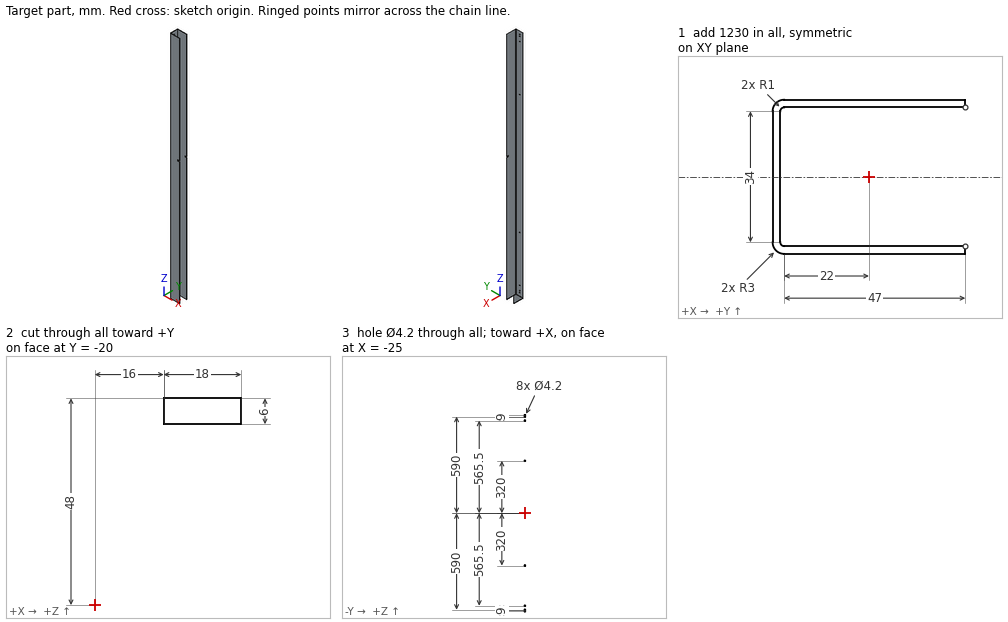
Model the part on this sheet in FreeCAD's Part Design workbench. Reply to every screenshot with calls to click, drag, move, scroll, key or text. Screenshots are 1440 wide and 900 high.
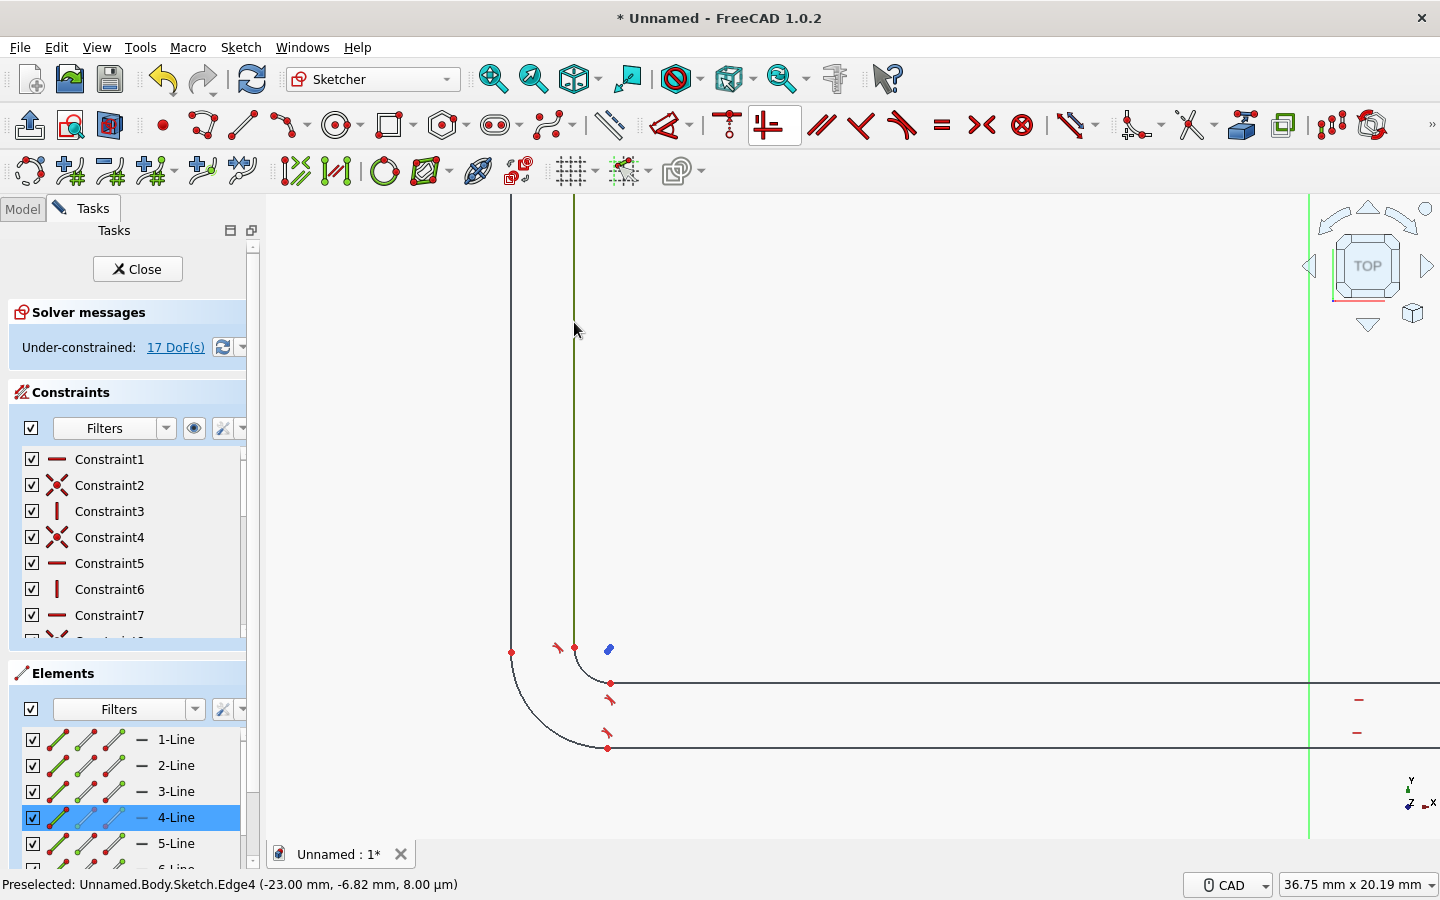
scroll(558, 694, down, 6)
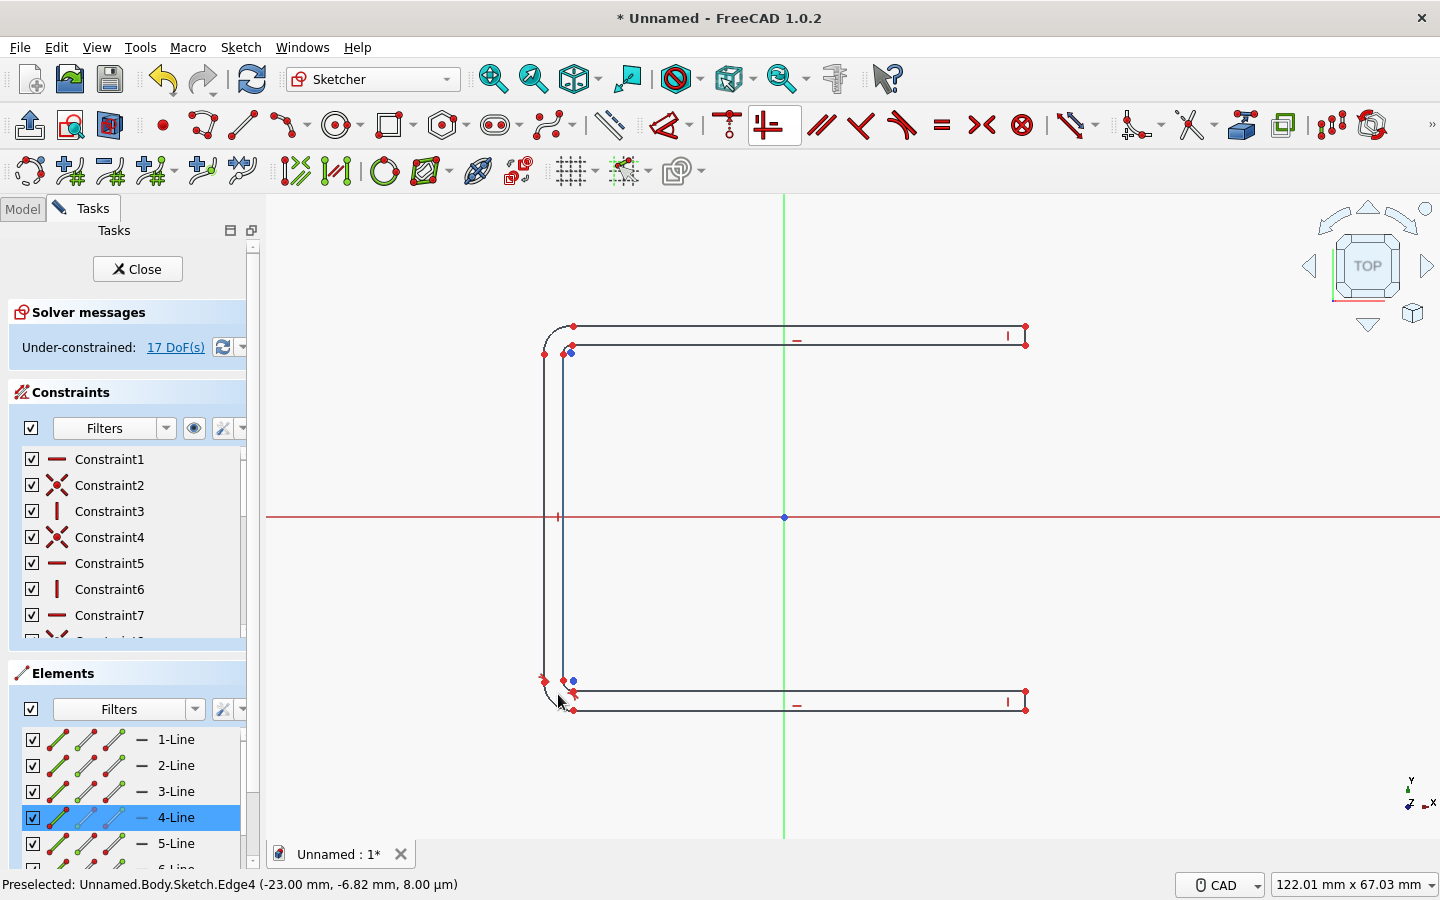
scroll(568, 346, up, 6)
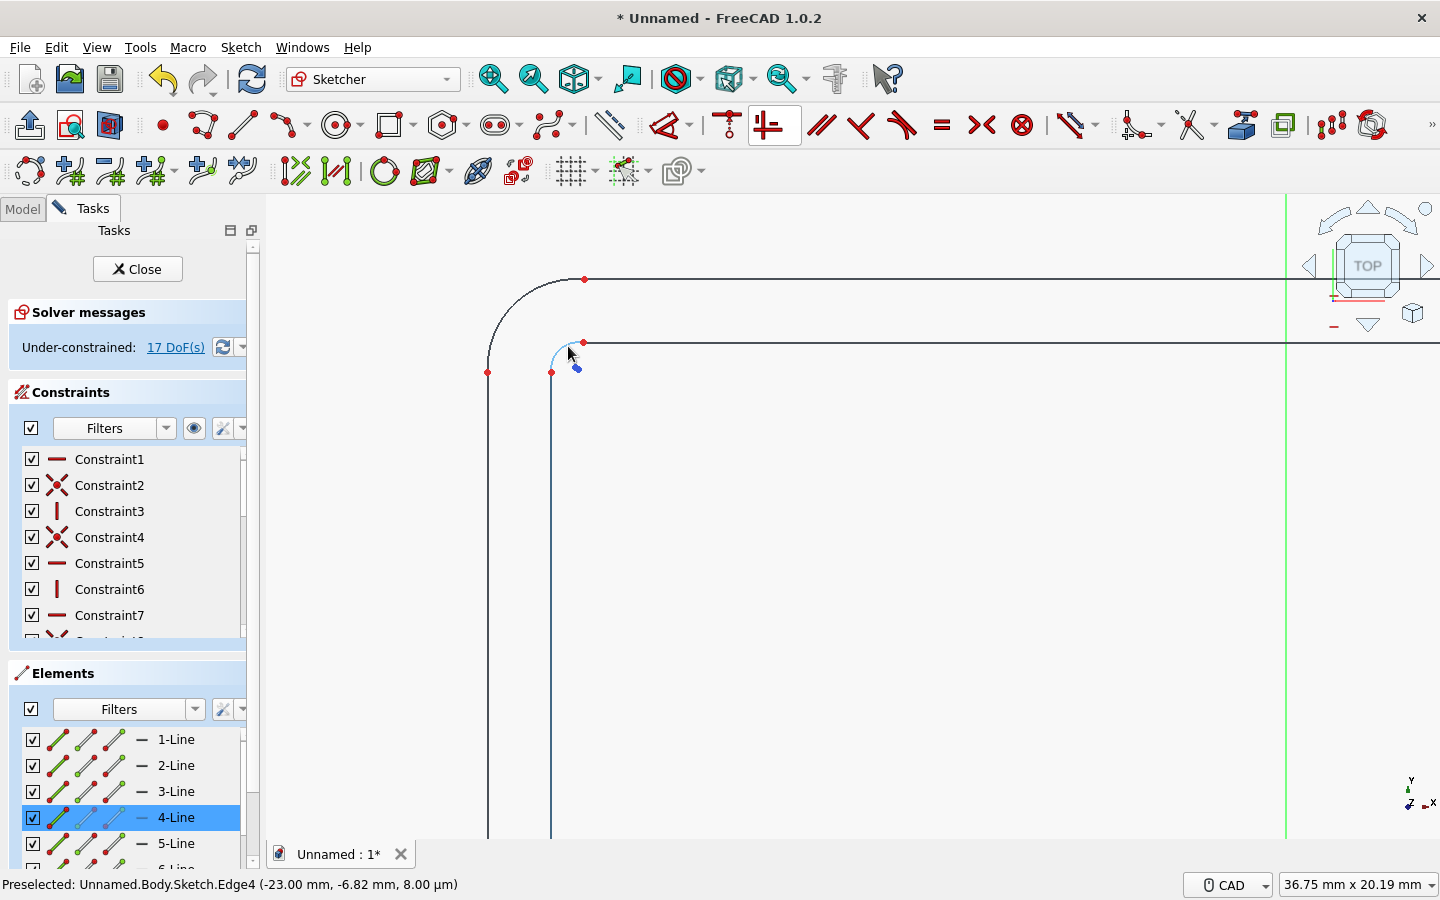
click(569, 344)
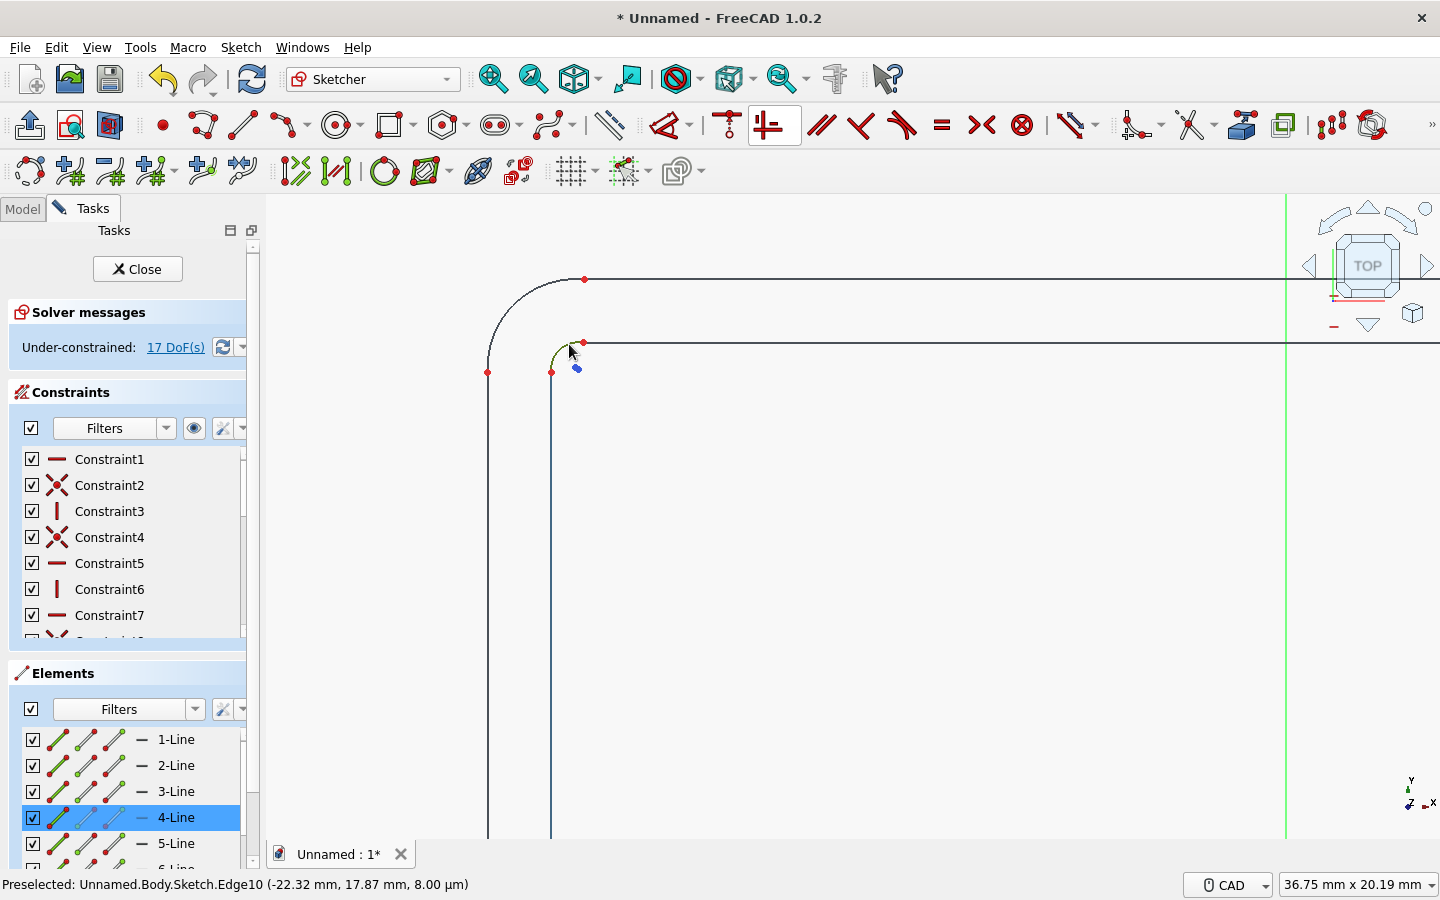
key(t)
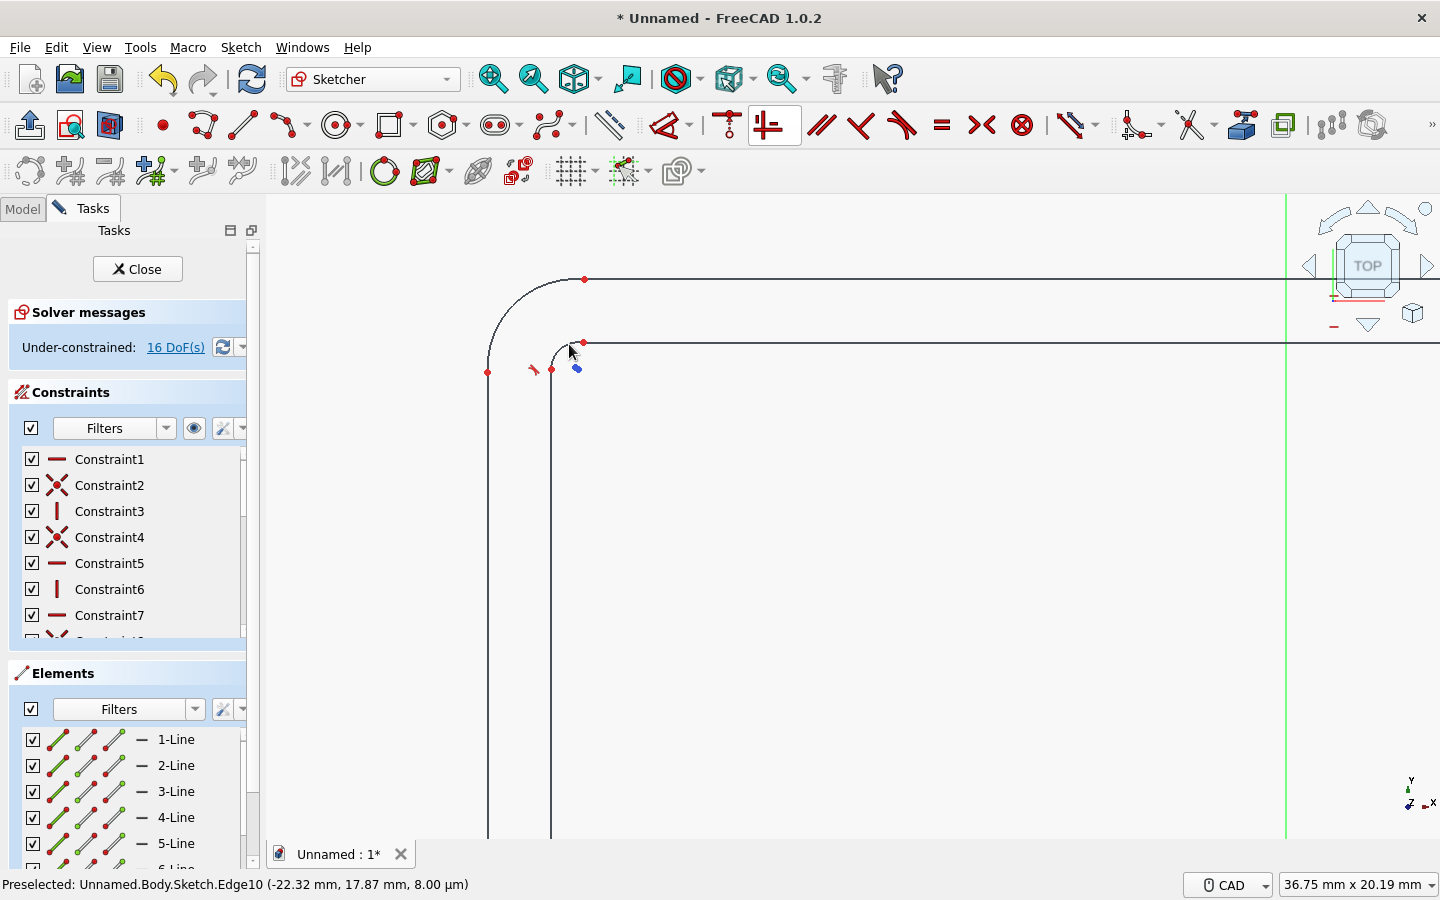
click(1034, 343)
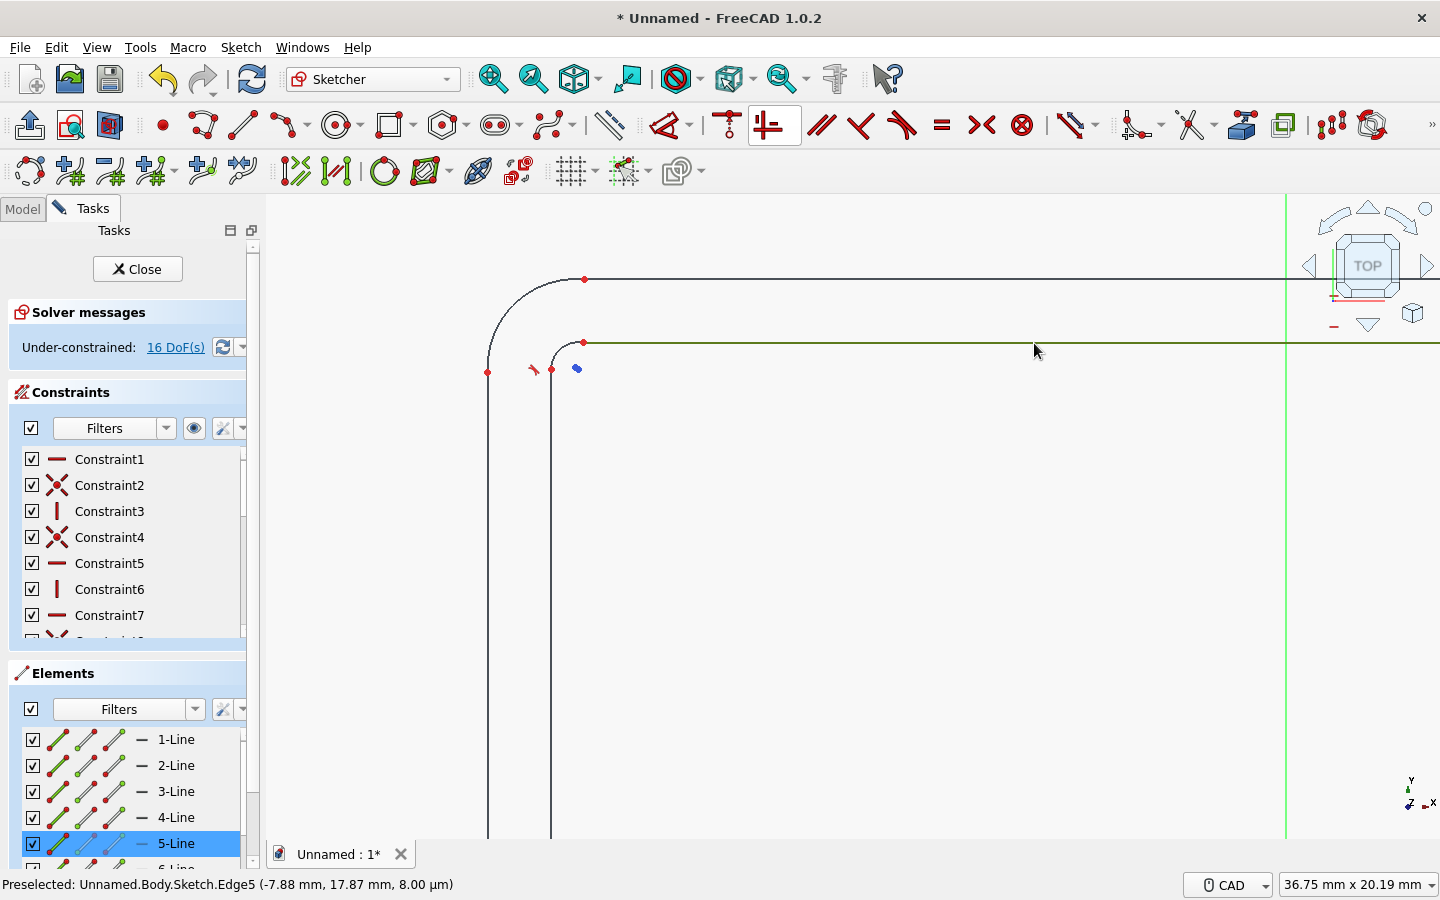
click(570, 344)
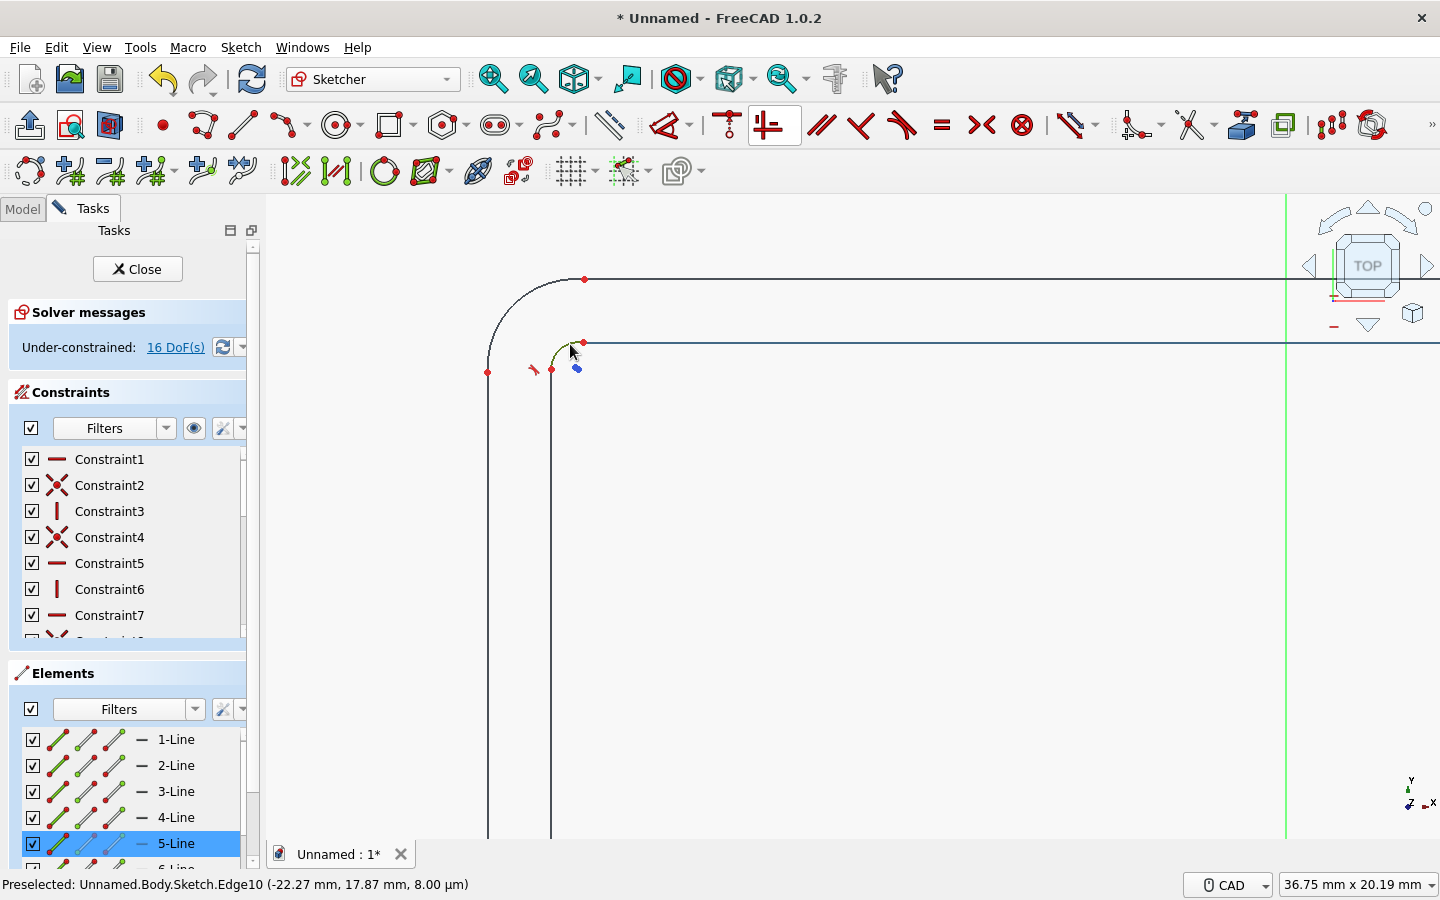
key(t)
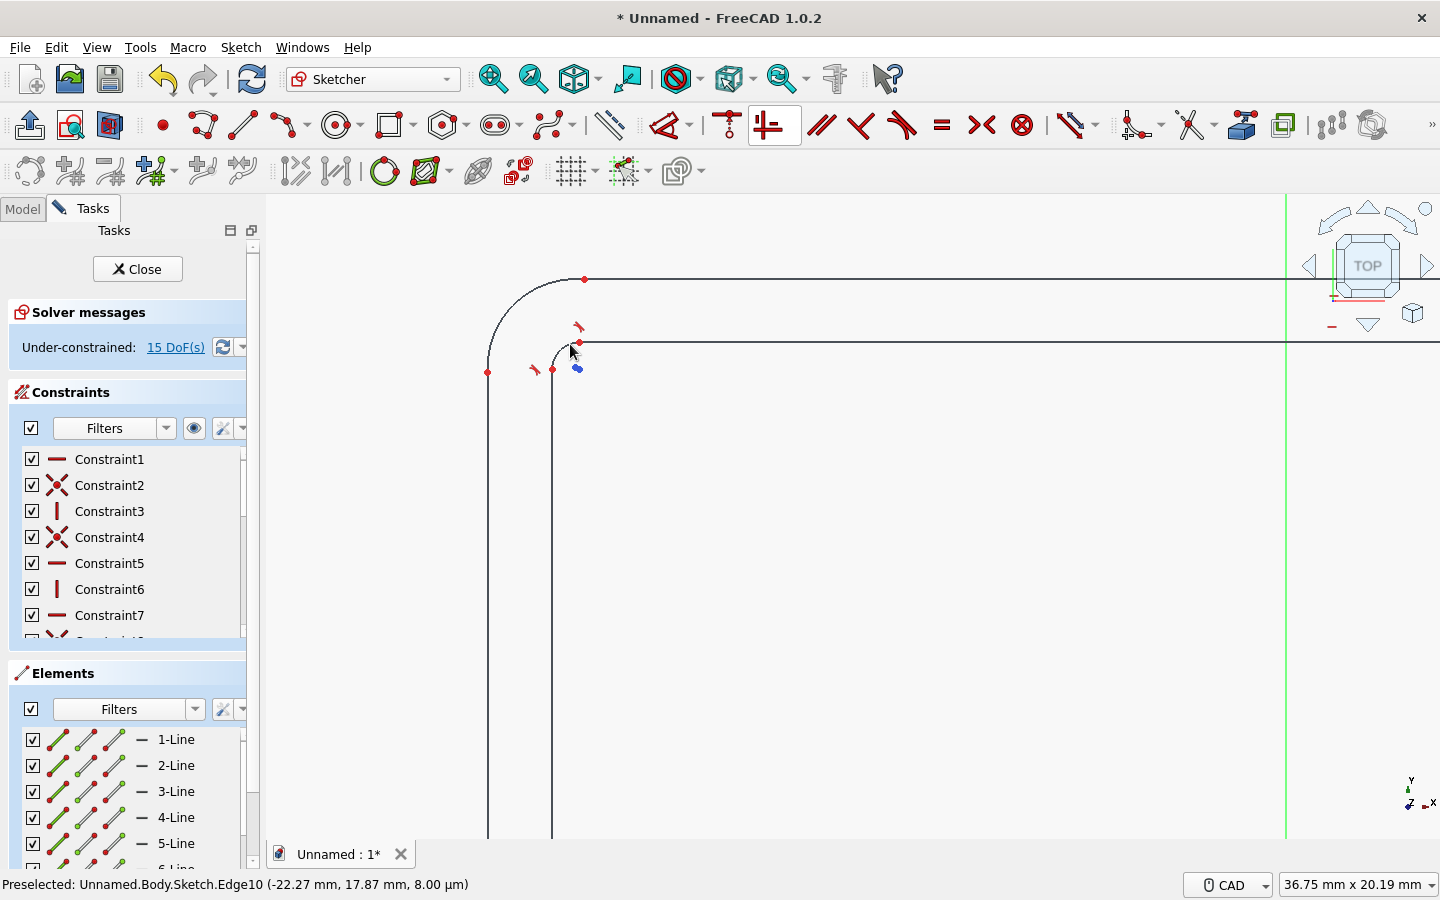
click(1034, 279)